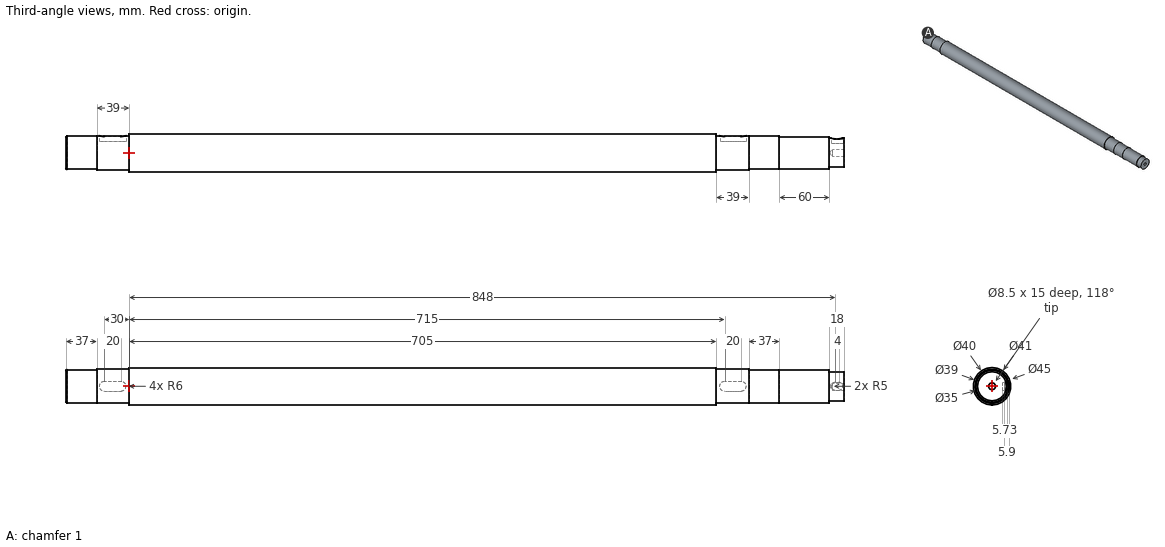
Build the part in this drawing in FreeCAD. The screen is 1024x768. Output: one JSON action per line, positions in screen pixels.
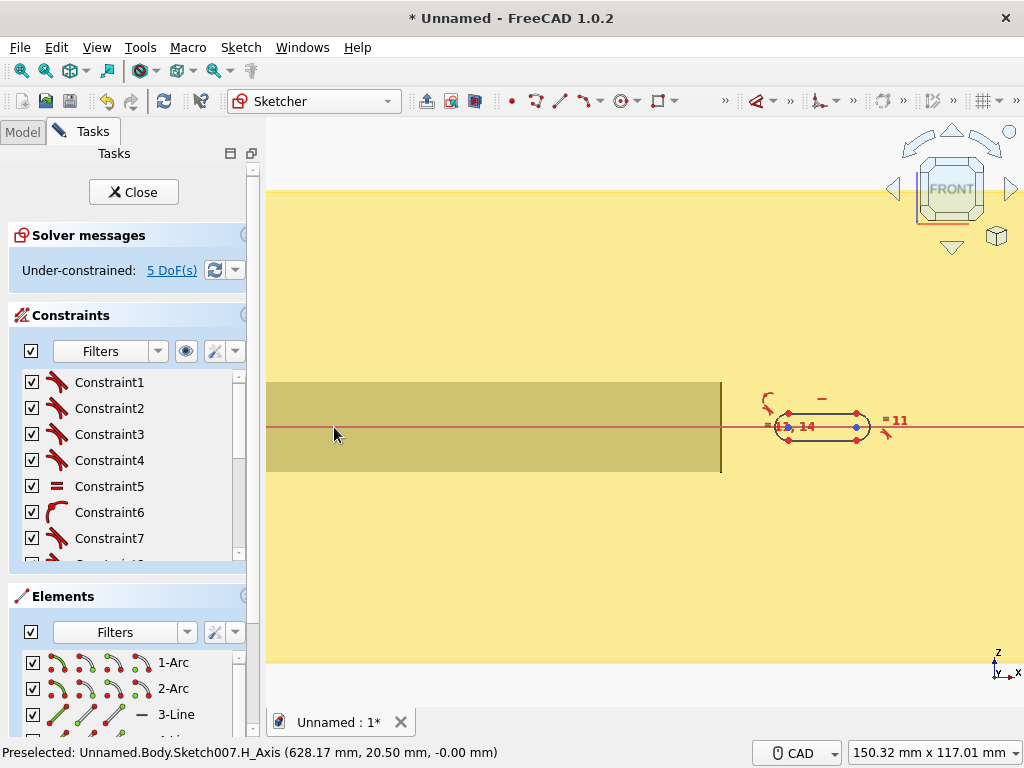
{"action": "scroll", "coordinate": [780, 410], "scroll_direction": "down", "scroll_amount": 11}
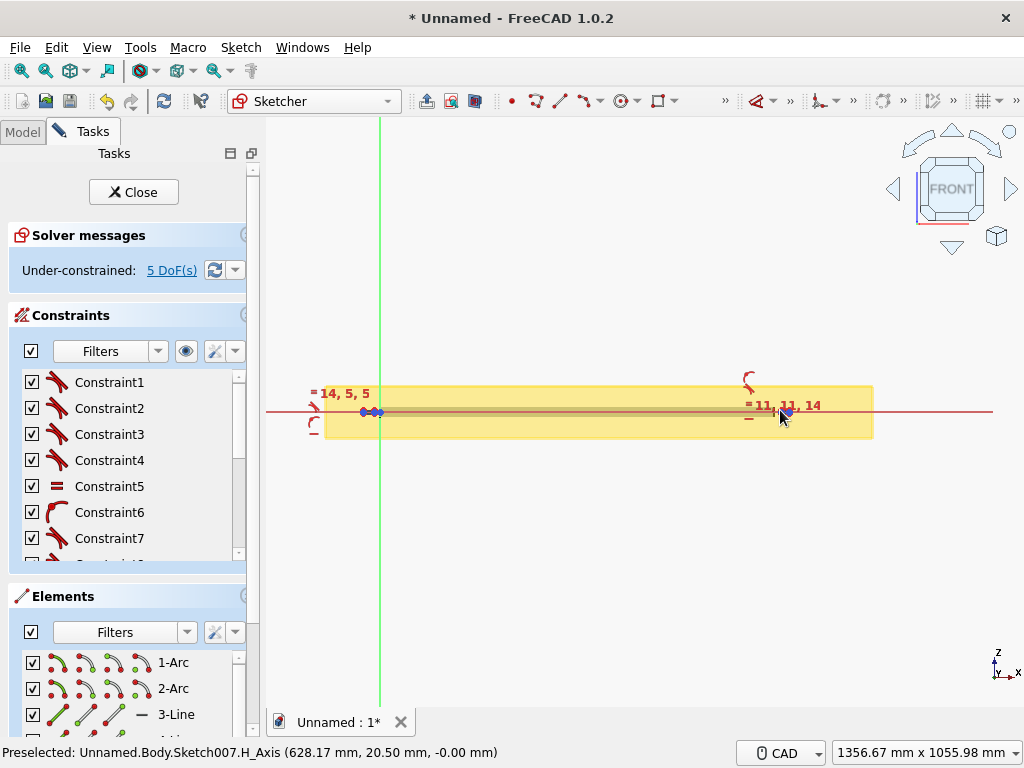
{"action": "scroll", "coordinate": [362, 412], "scroll_direction": "up", "scroll_amount": 13}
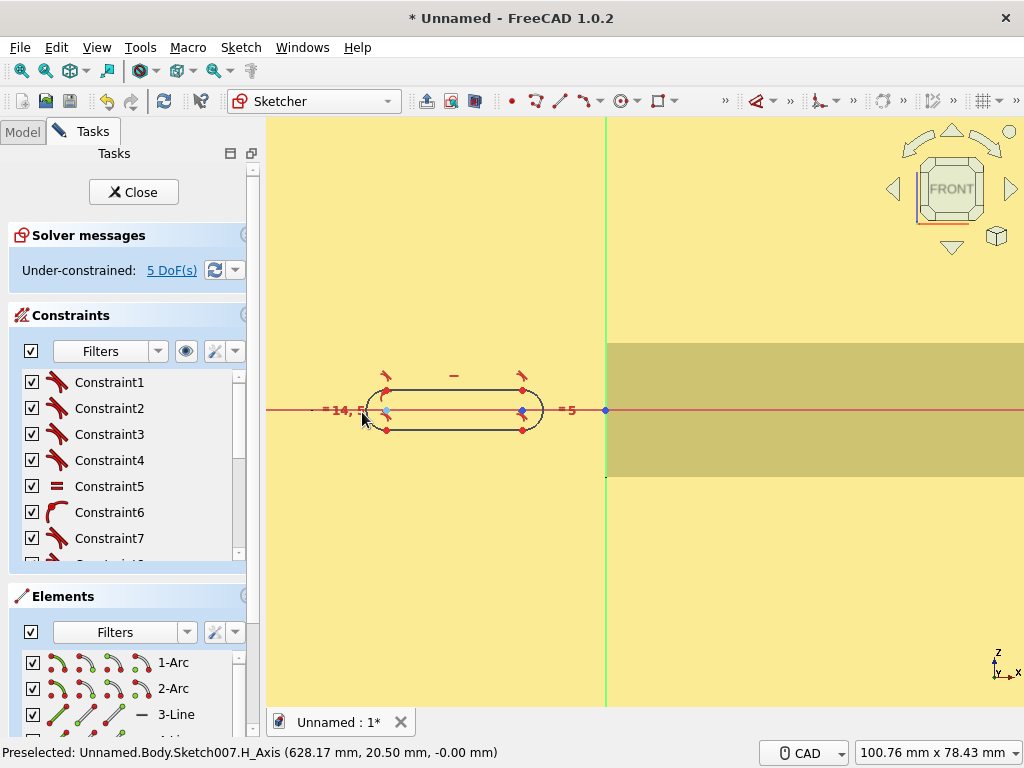
{"action": "left_click", "coordinate": [366, 410]}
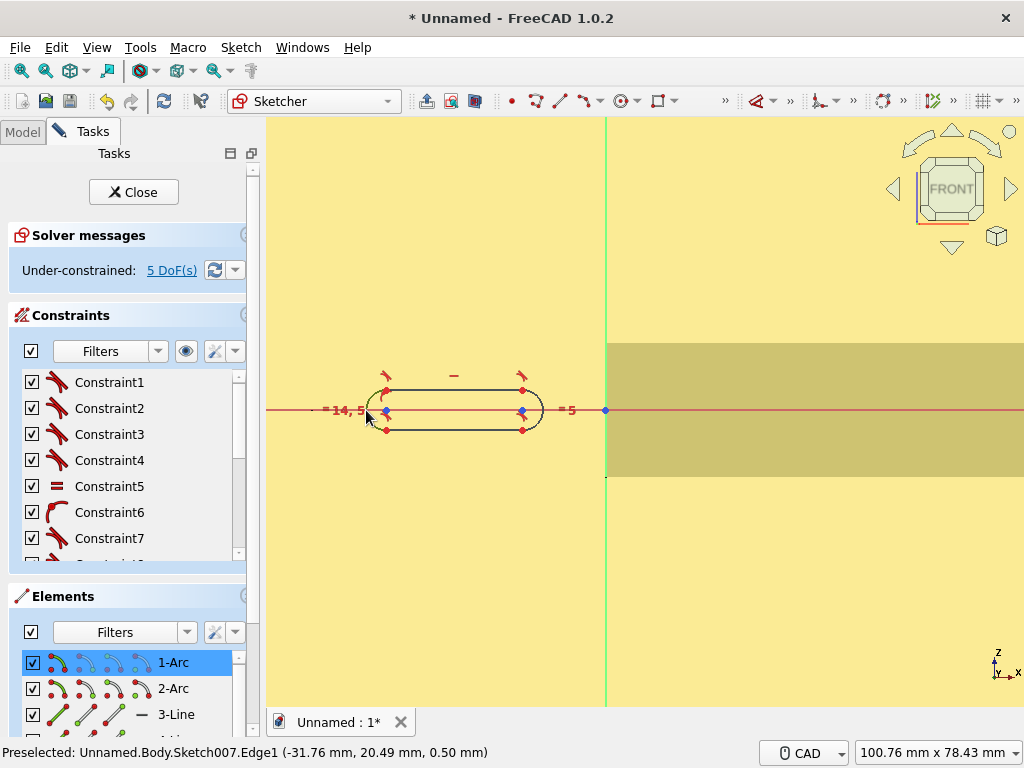
{"action": "left_click", "coordinate": [776, 102]}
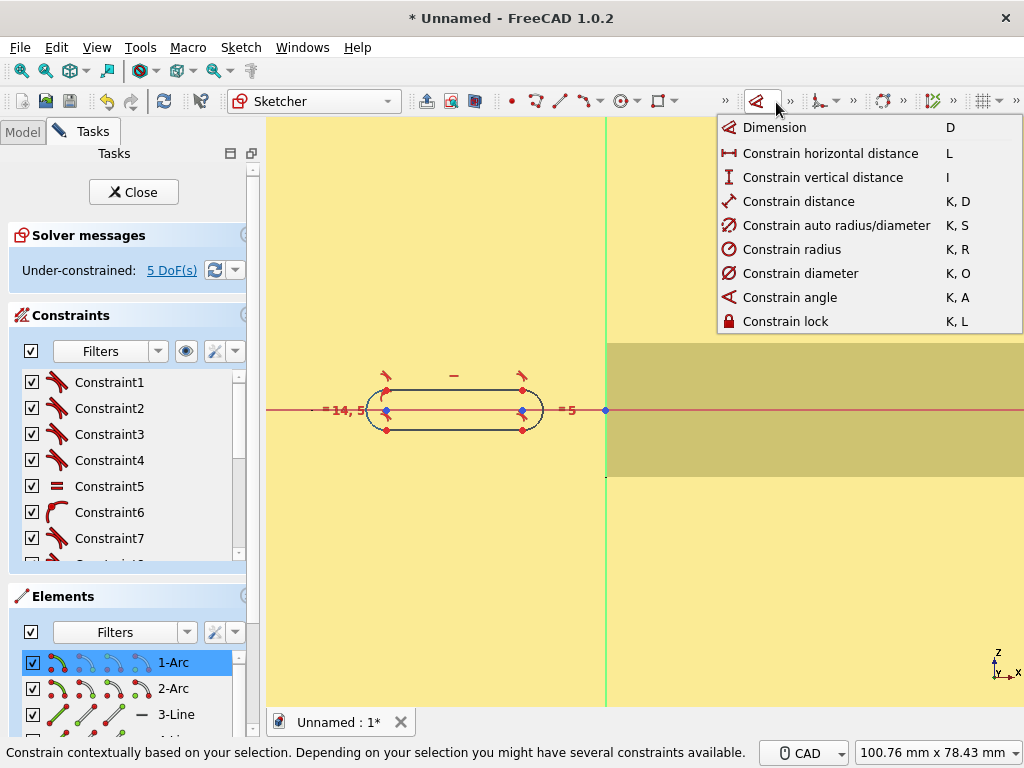
{"action": "left_click", "coordinate": [870, 249]}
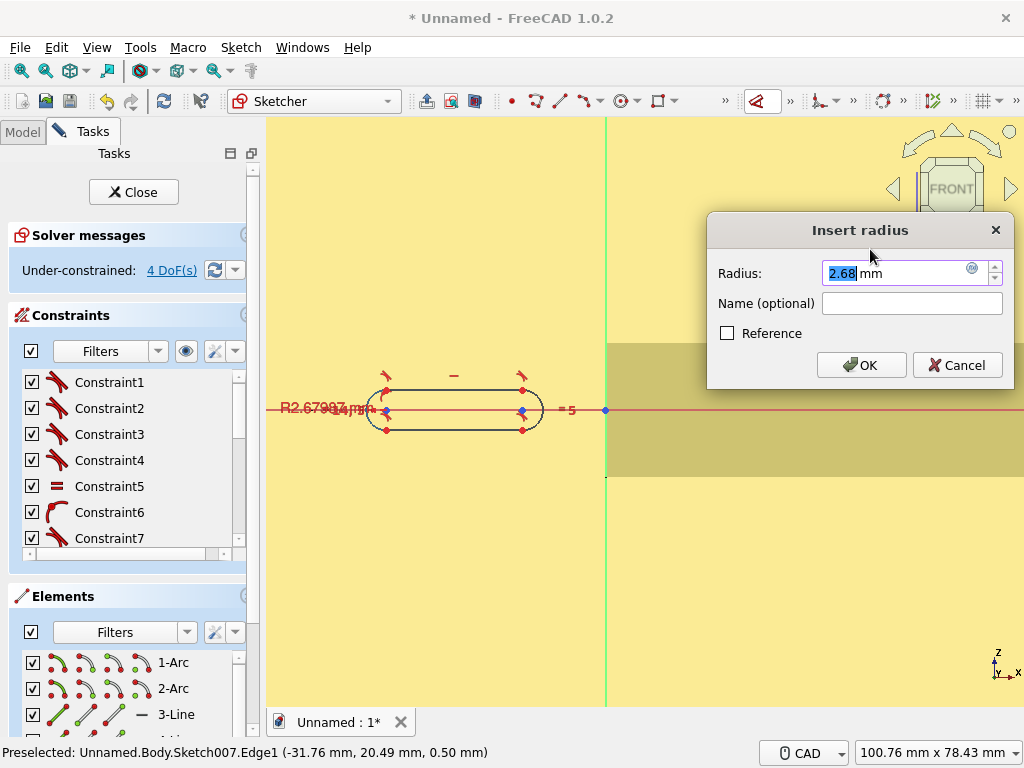
{"action": "type", "text": "6"}
{"action": "key", "text": "Return"}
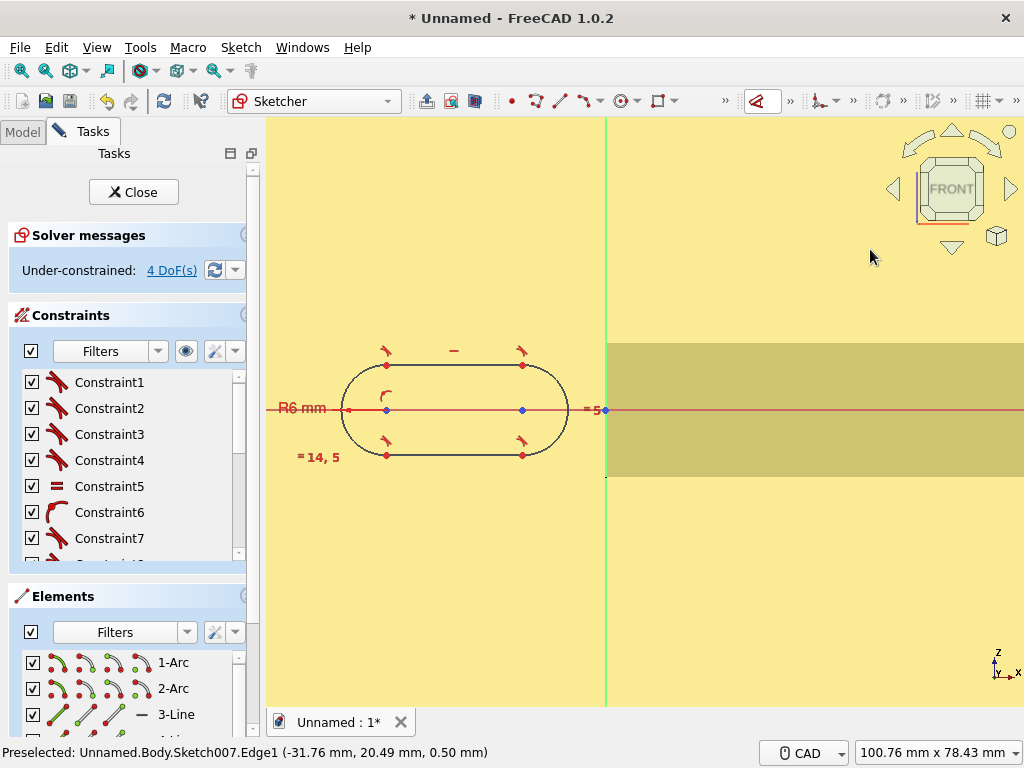
{"action": "scroll", "coordinate": [361, 412], "scroll_direction": "down", "scroll_amount": 13}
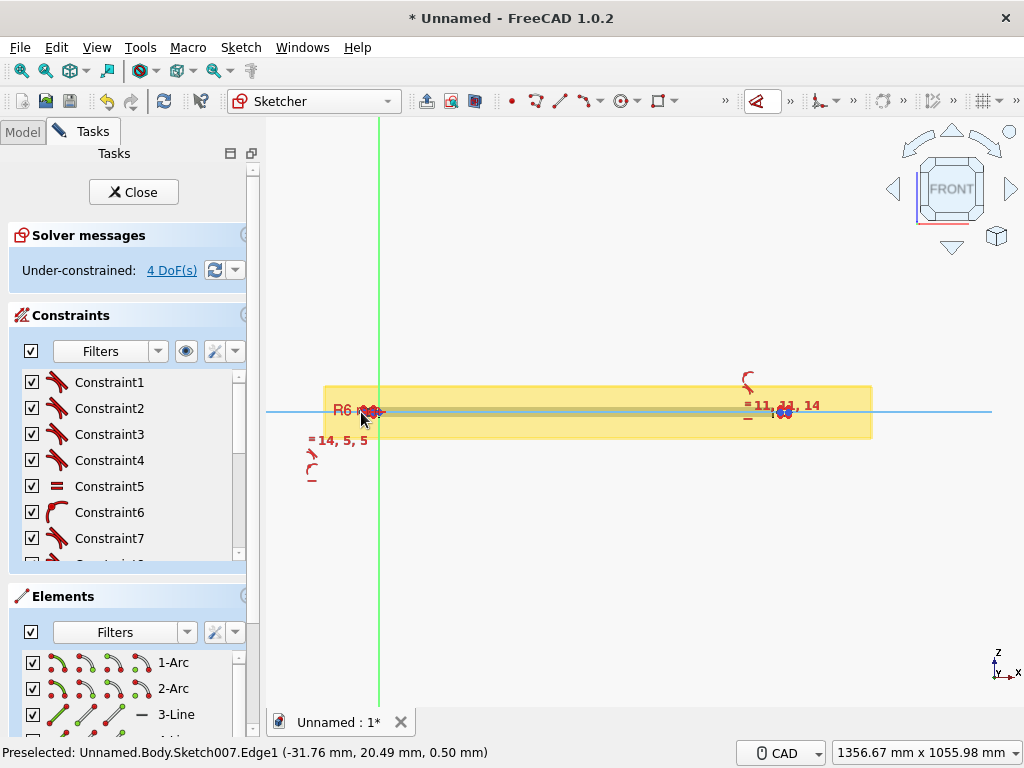
{"action": "scroll", "coordinate": [366, 409], "scroll_direction": "up", "scroll_amount": 8}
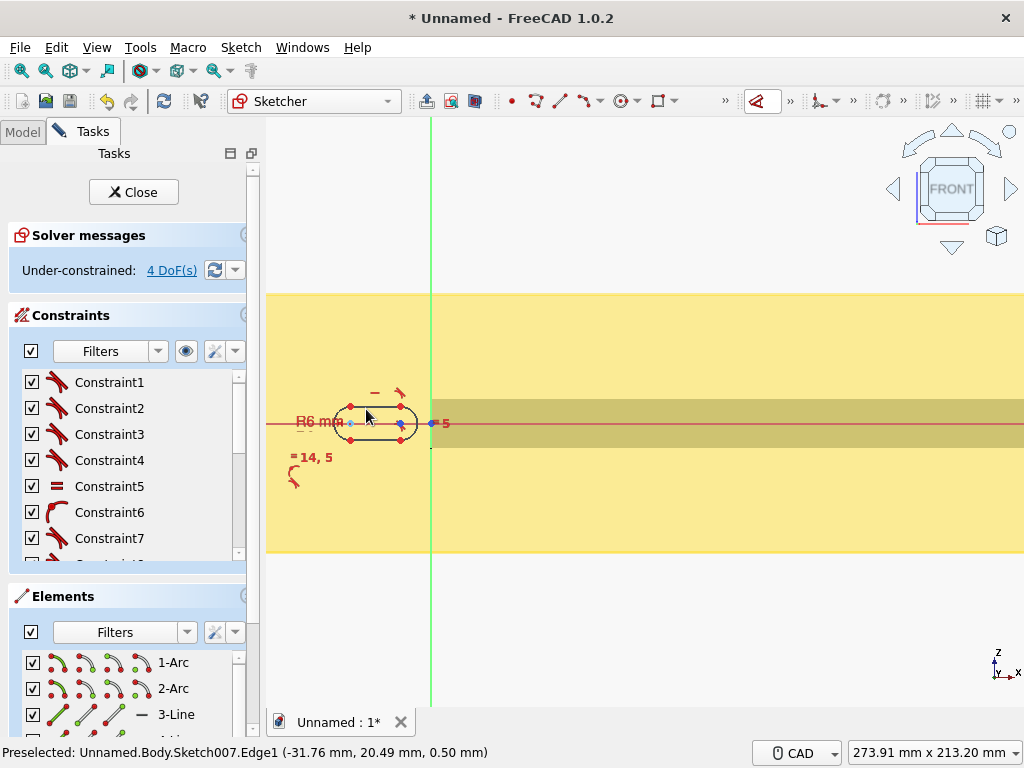
{"action": "left_click", "coordinate": [366, 407]}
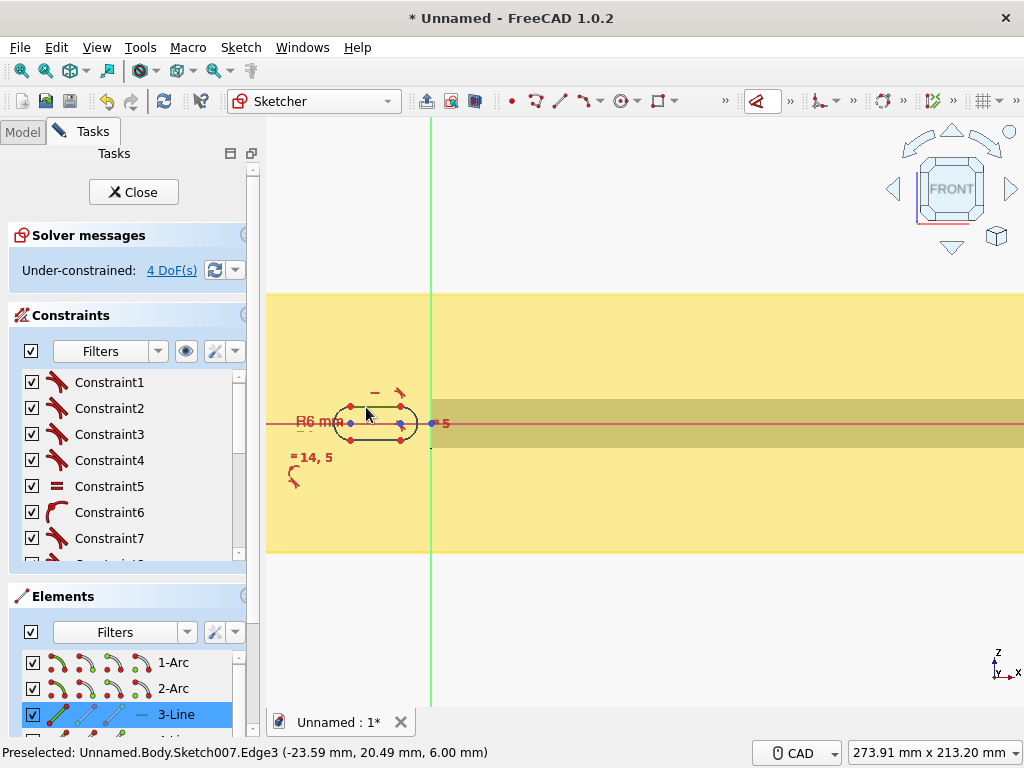
{"action": "left_click", "coordinate": [776, 102]}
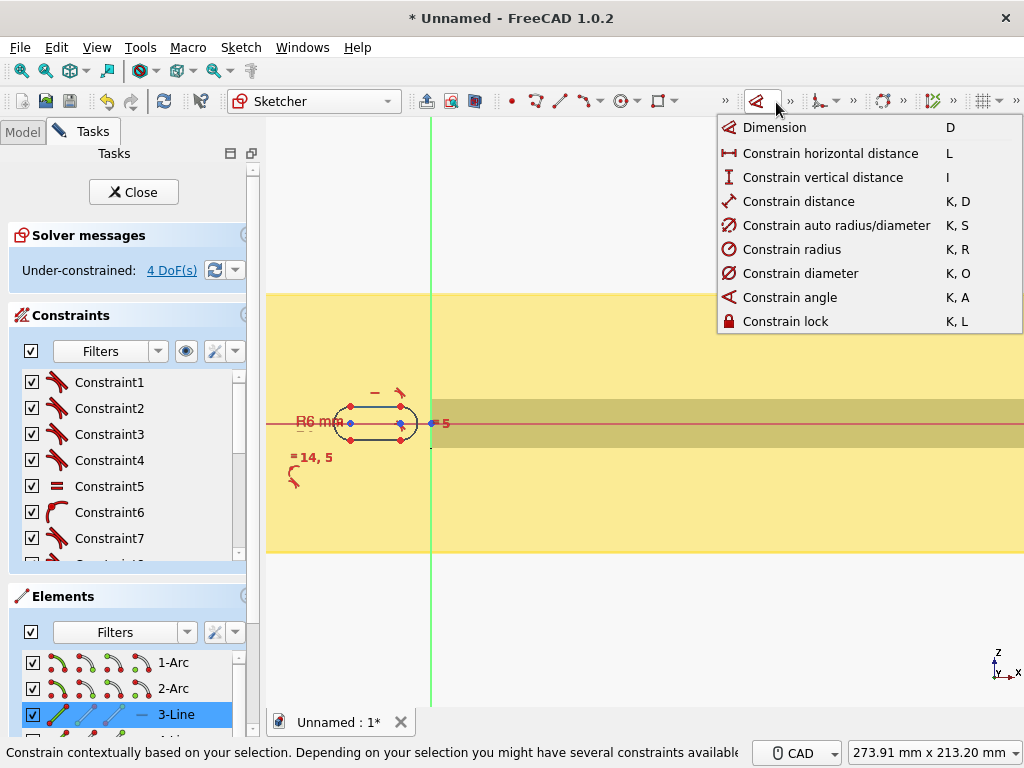
{"action": "left_click", "coordinate": [870, 153]}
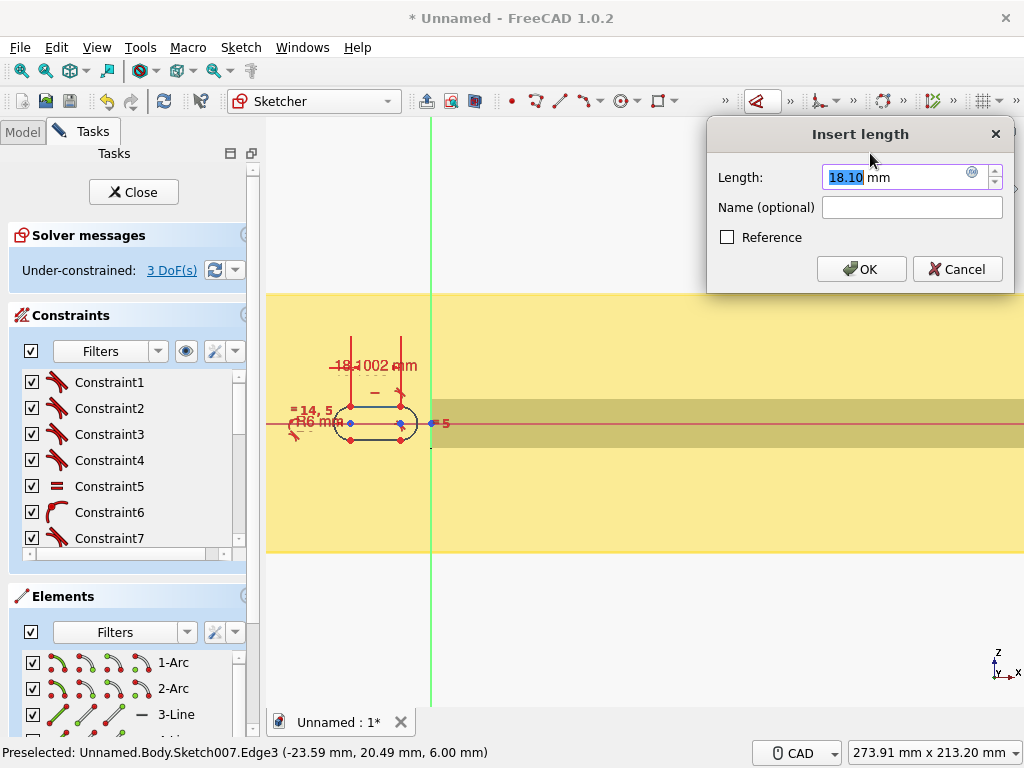
{"action": "type", "text": "20"}
{"action": "key", "text": "Return"}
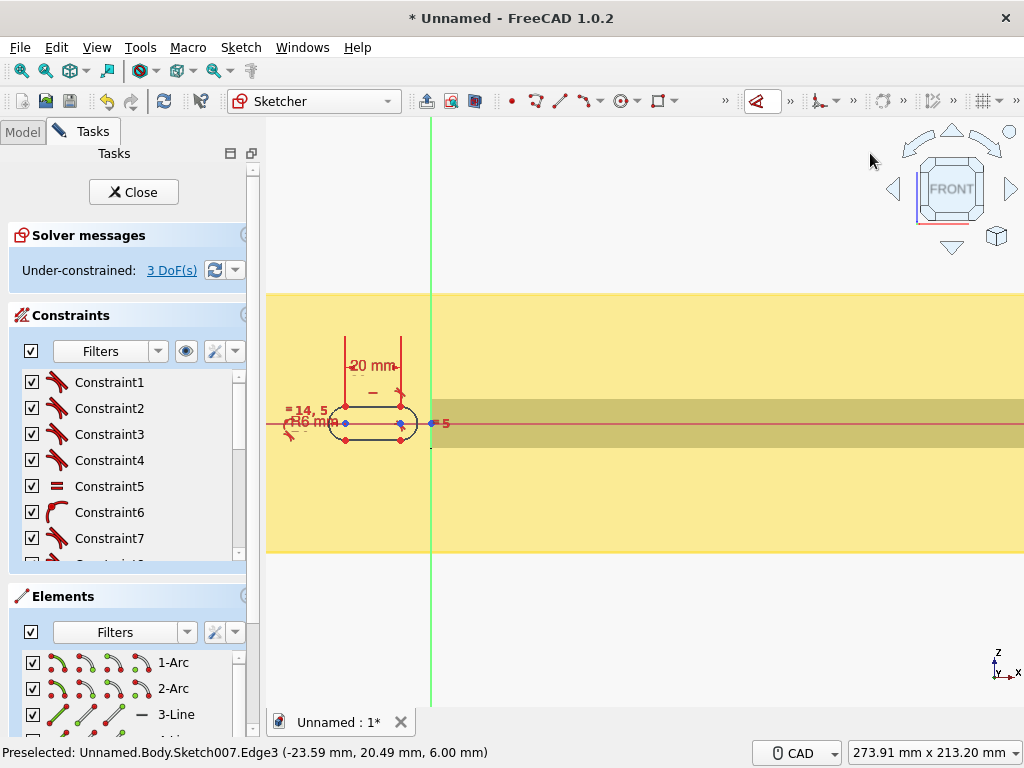
{"action": "scroll", "coordinate": [366, 409], "scroll_direction": "down", "scroll_amount": 8}